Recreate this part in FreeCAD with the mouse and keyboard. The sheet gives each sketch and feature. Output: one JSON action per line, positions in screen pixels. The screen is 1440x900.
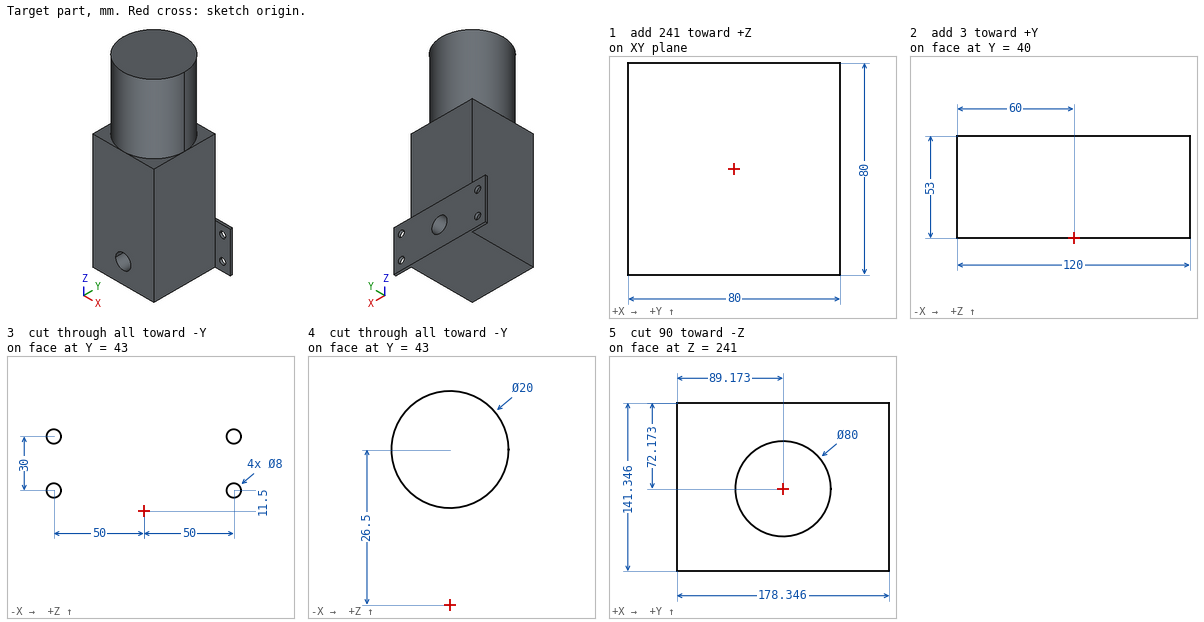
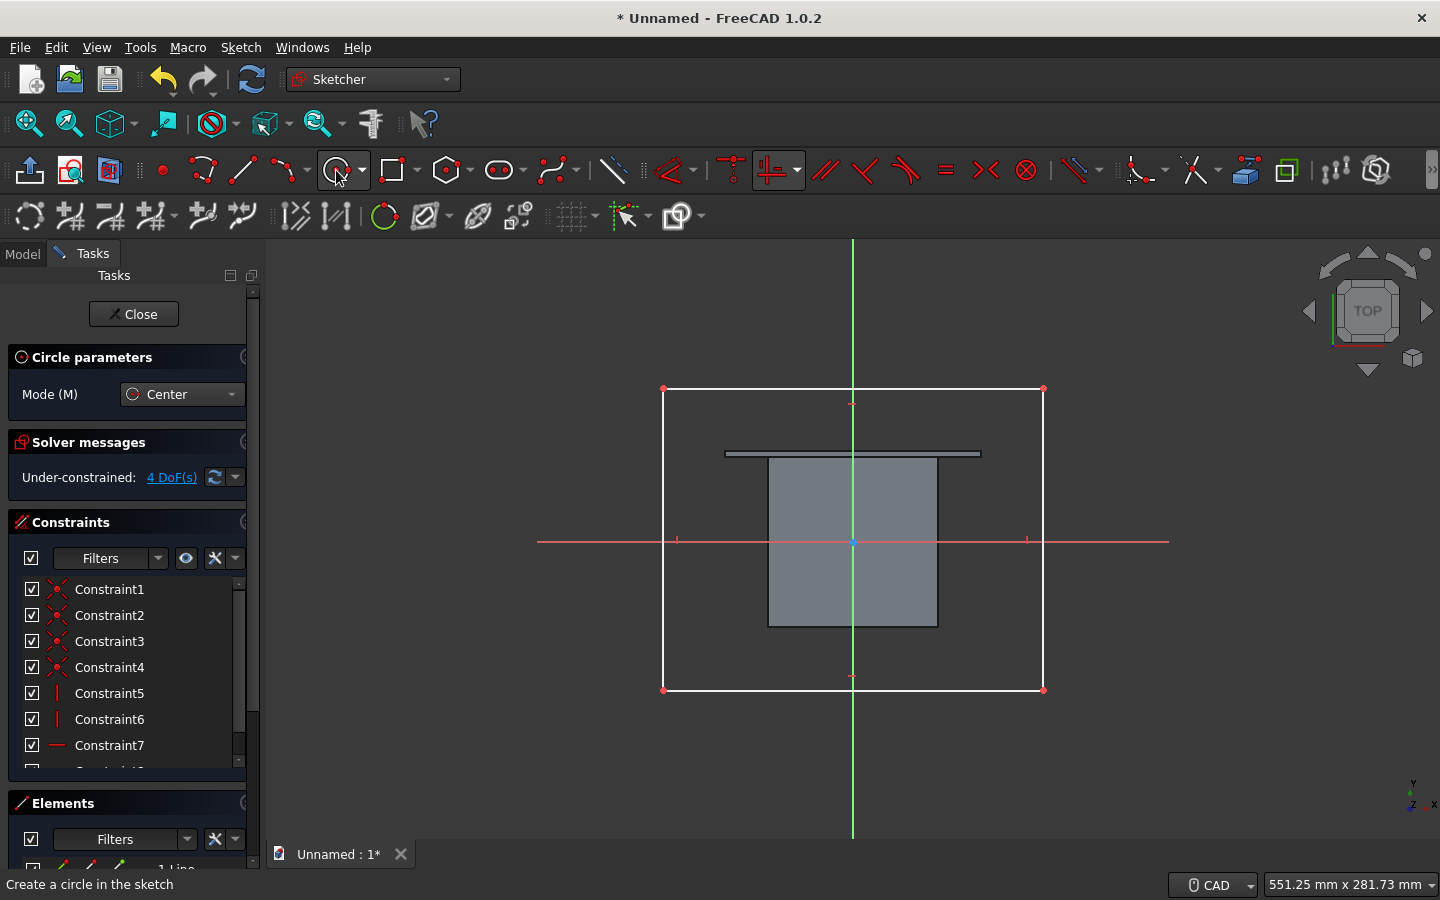
{"action": "left_click", "coordinate": [853, 542]}
{"action": "left_click", "coordinate": [913, 482]}
{"action": "key", "text": "Escape"}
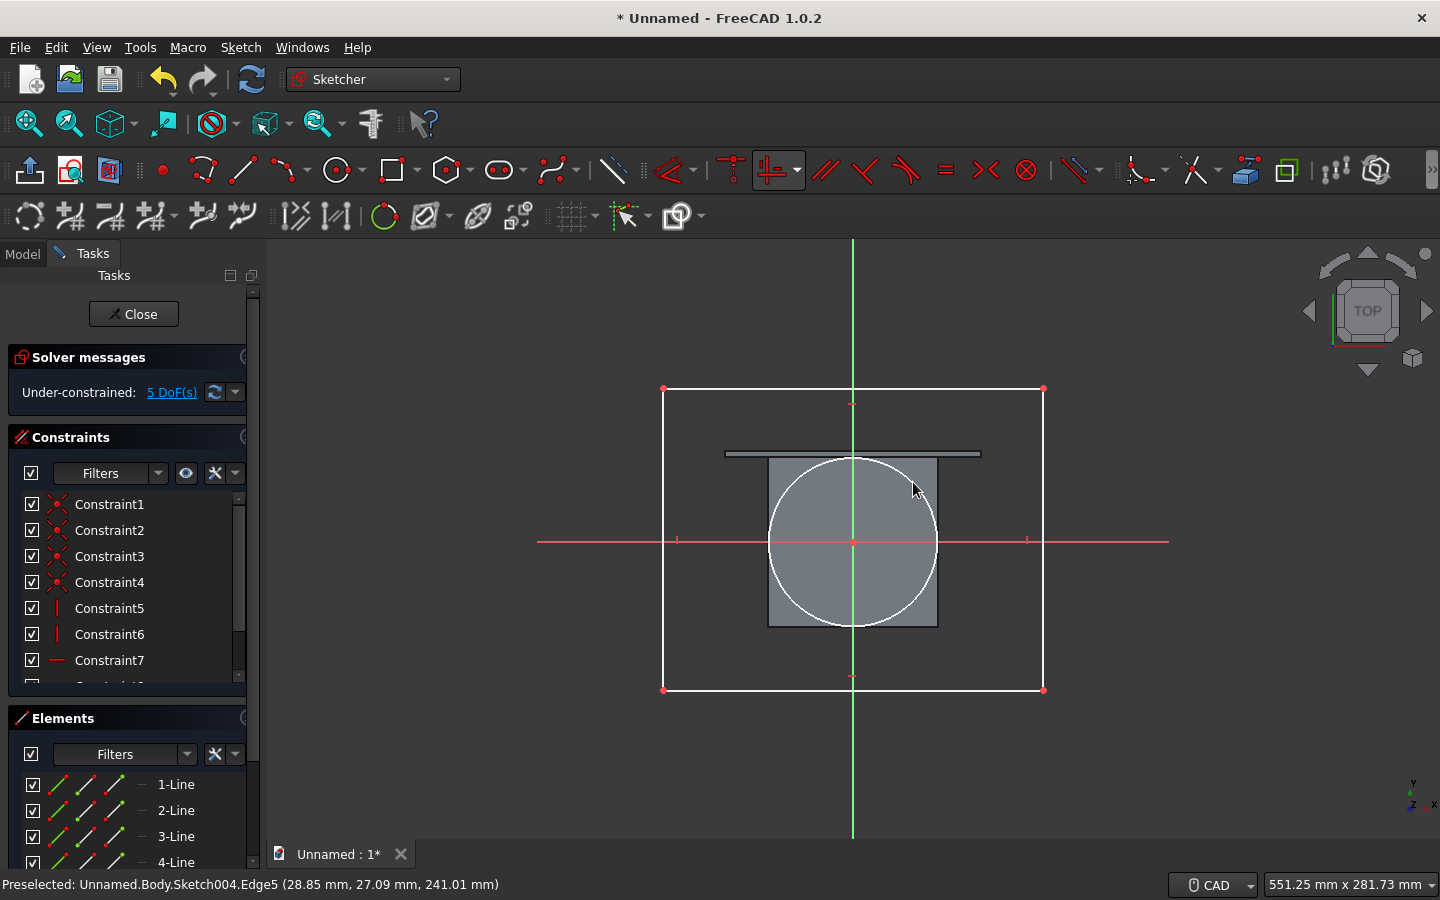
{"action": "left_click", "coordinate": [668, 170]}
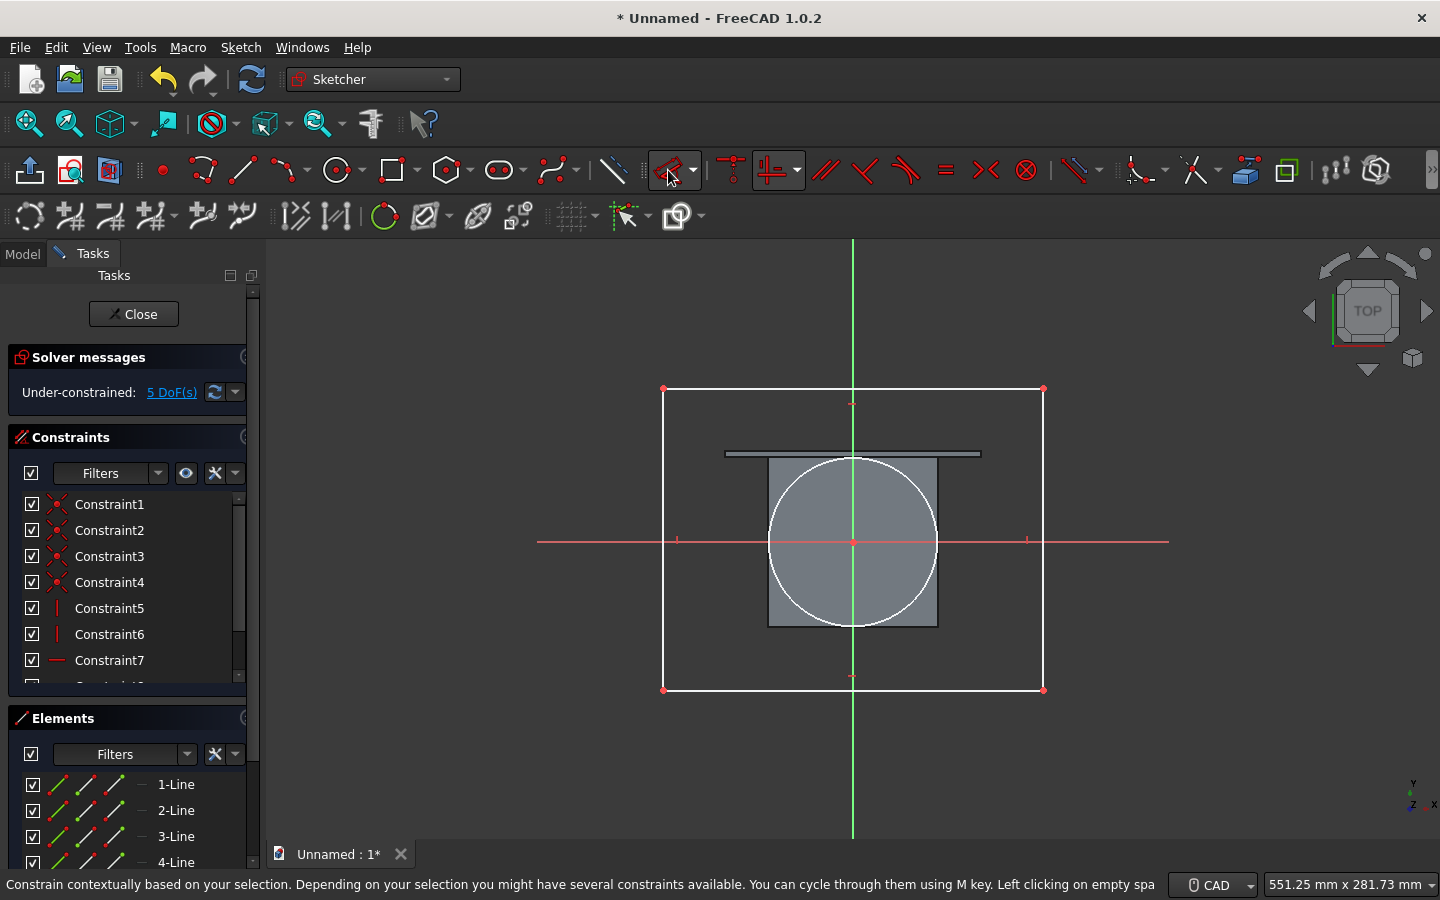
{"action": "left_click", "coordinate": [912, 482]}
{"action": "left_click", "coordinate": [934, 459]}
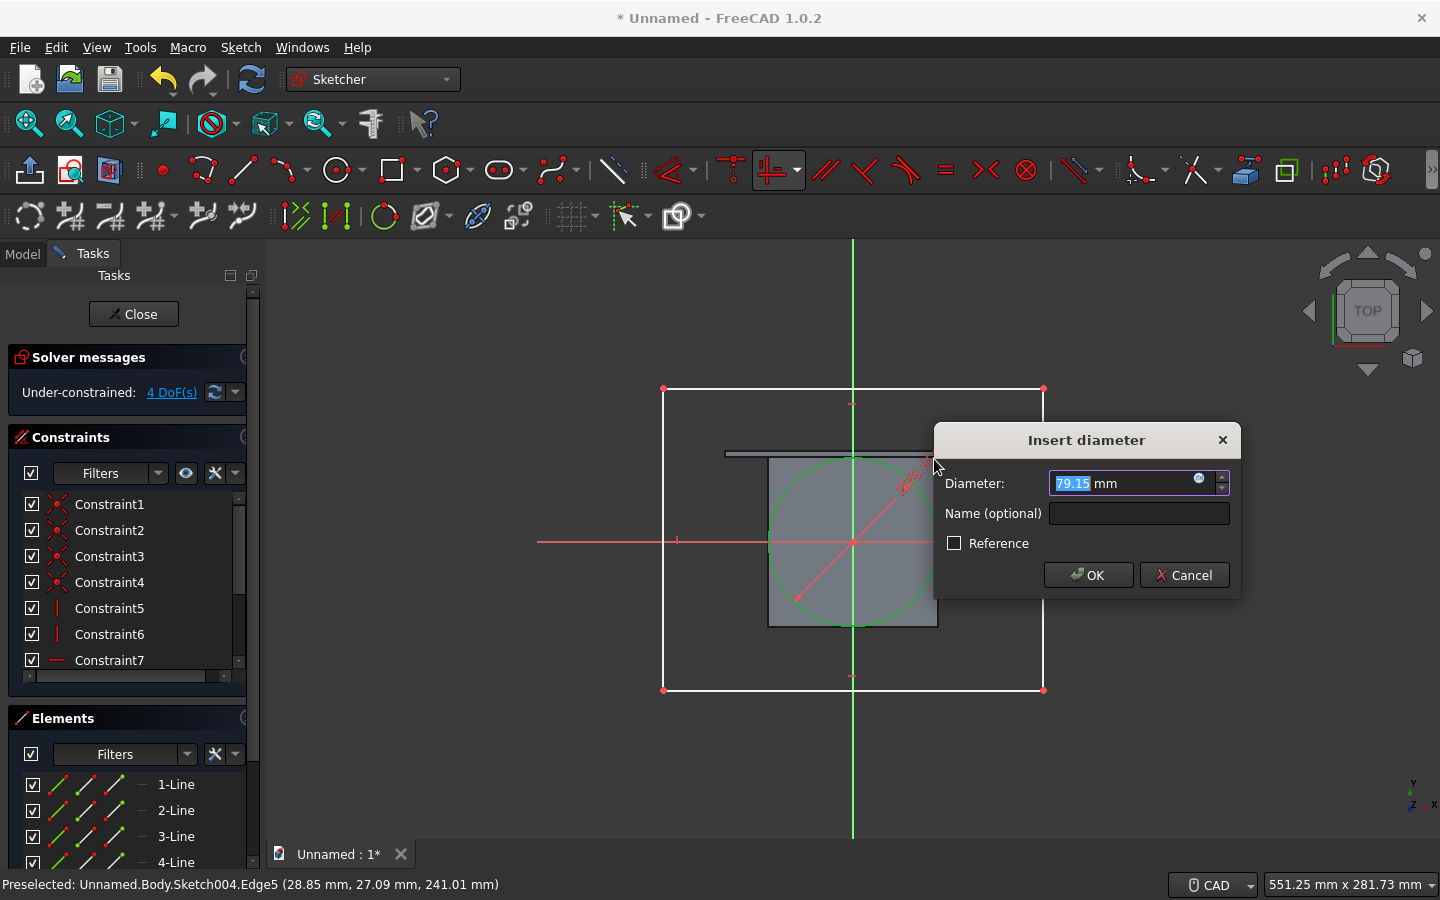
{"action": "type", "text": "80"}
{"action": "key", "text": "Return"}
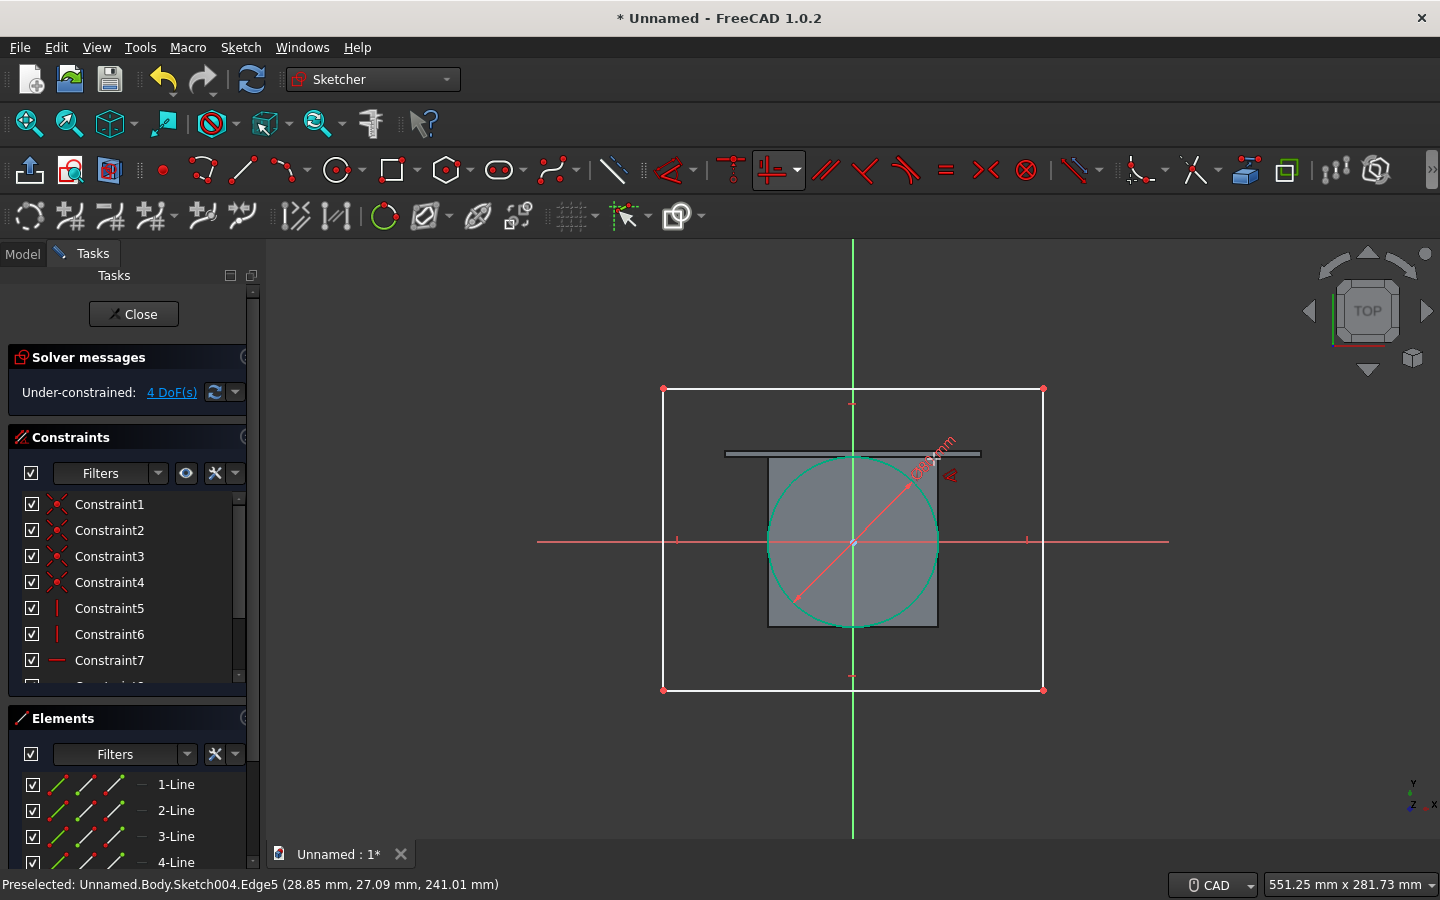
{"action": "left_click", "coordinate": [663, 480]}
{"action": "left_click", "coordinate": [629, 471]}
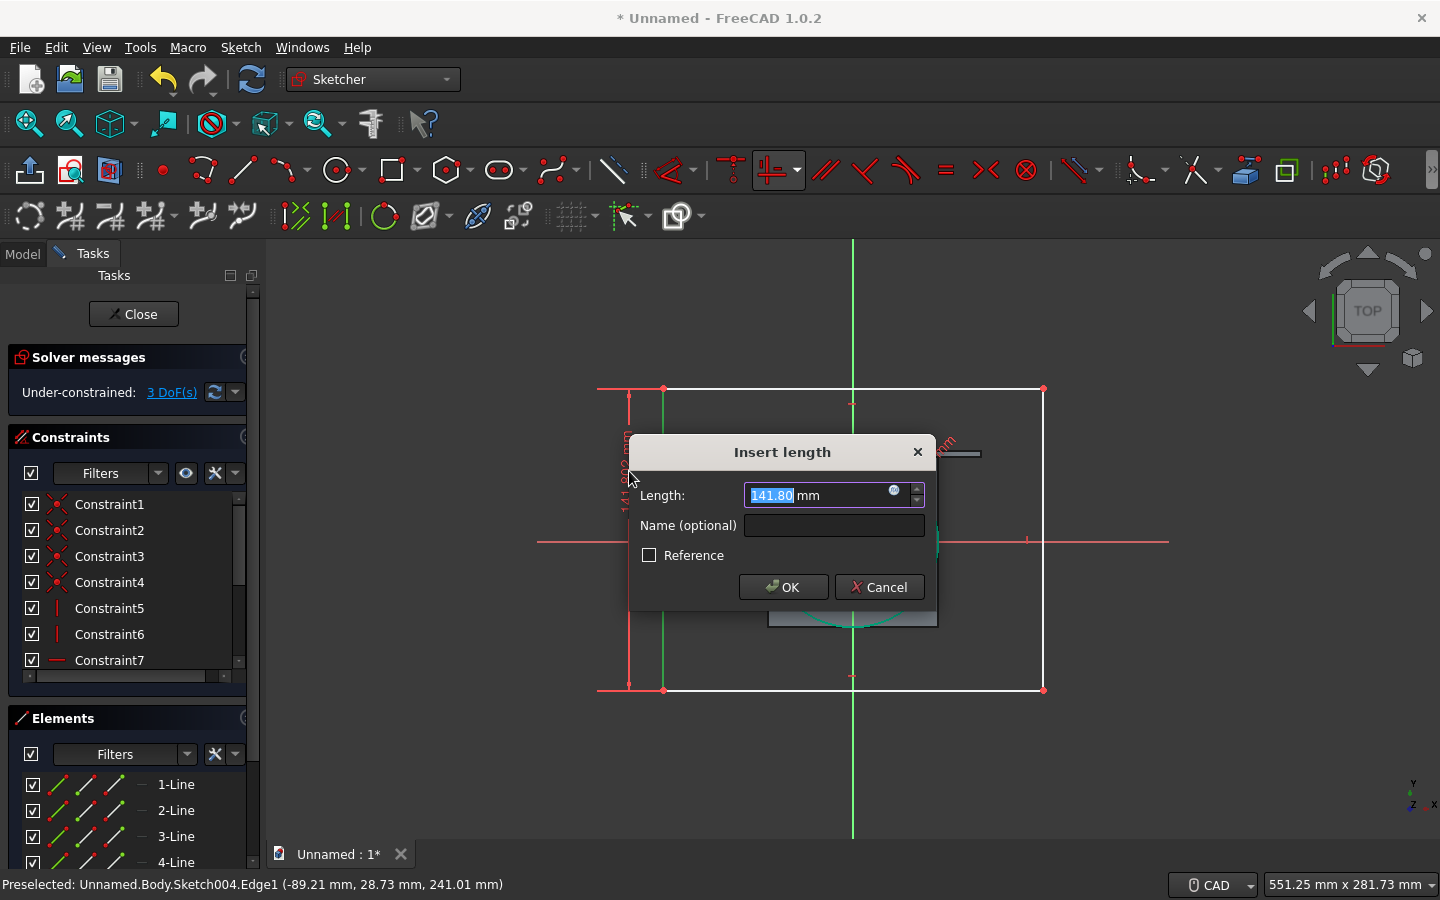
{"action": "type", "text": "141.346"}
{"action": "key", "text": "Return"}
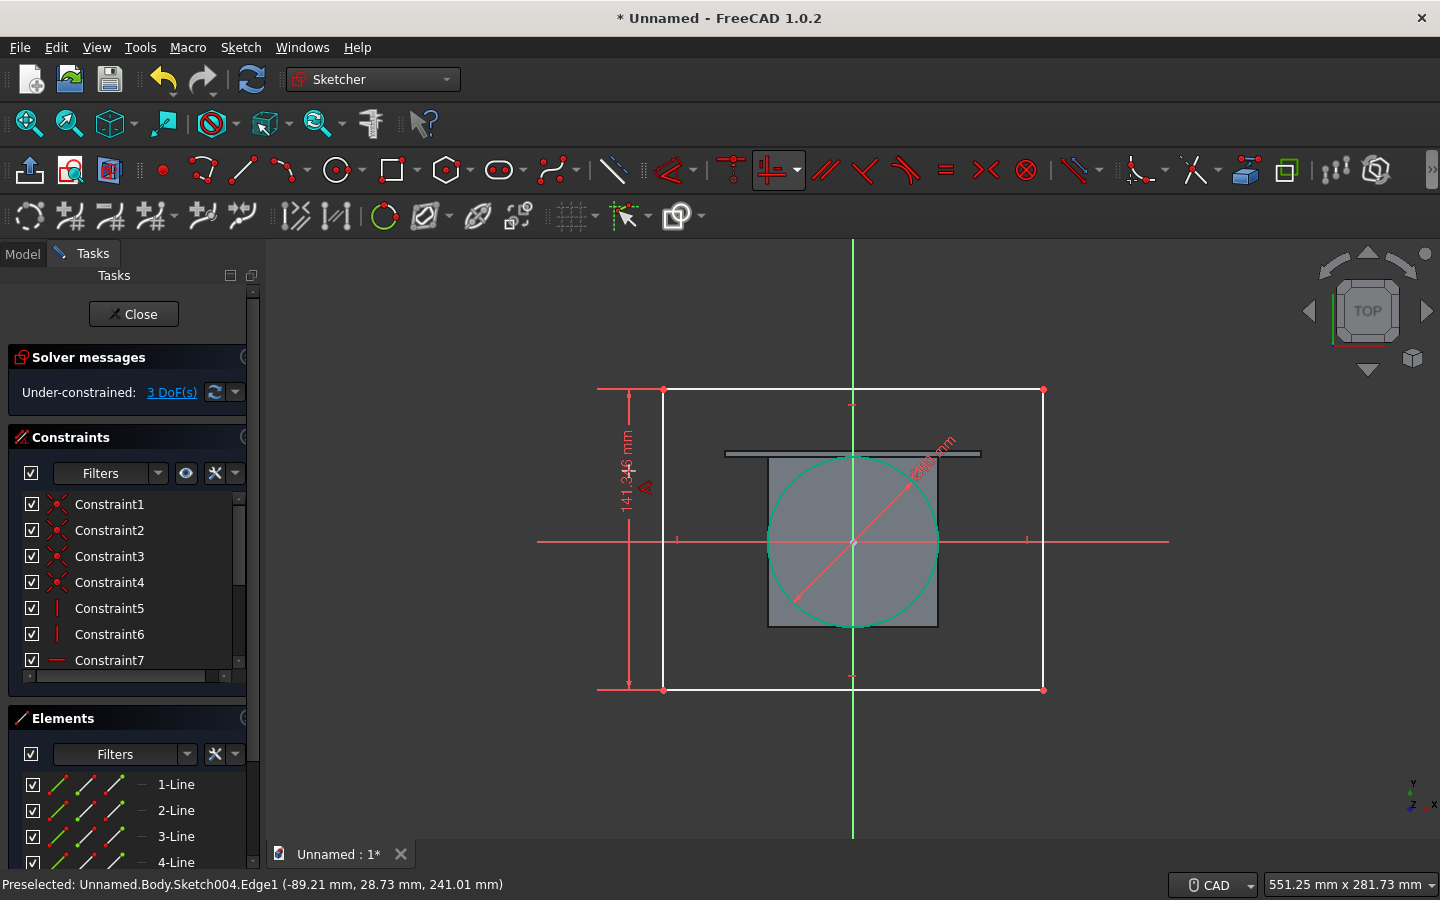
{"action": "left_click", "coordinate": [777, 690]}
{"action": "left_click", "coordinate": [766, 724]}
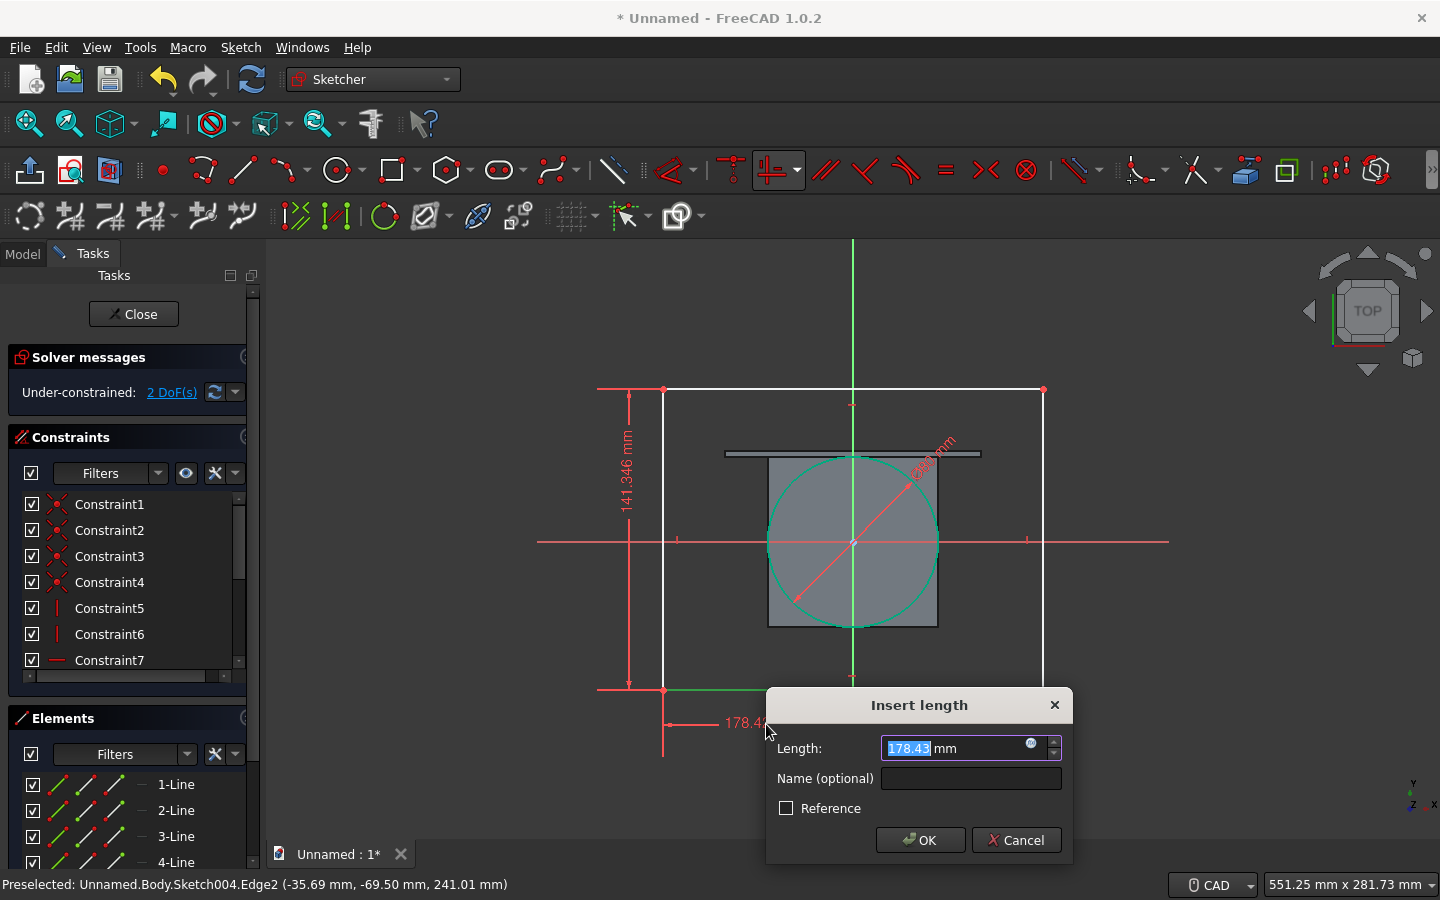
{"action": "type", "text": "178.346"}
{"action": "key", "text": "Return"}